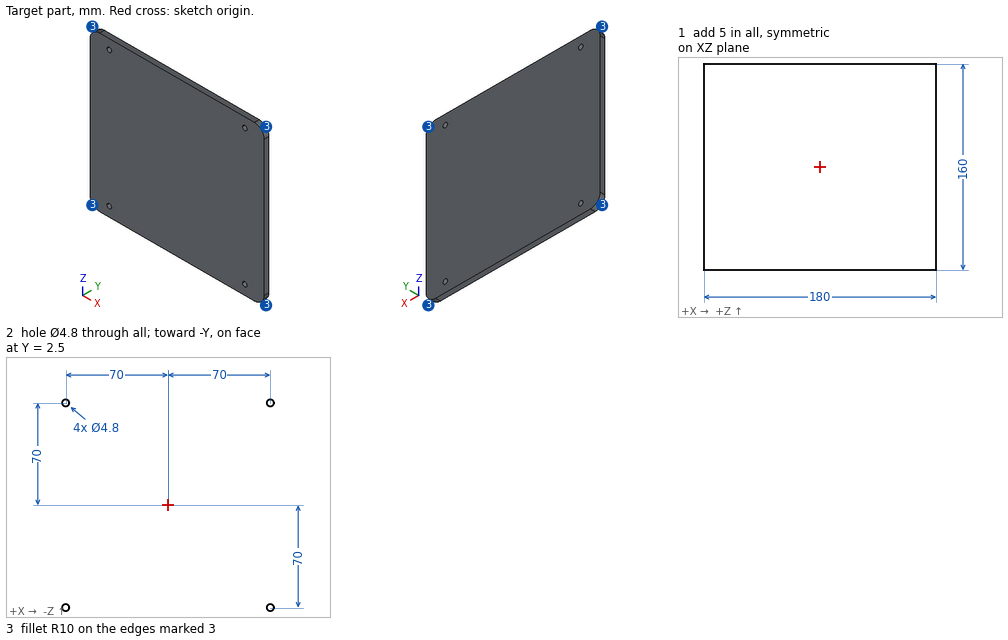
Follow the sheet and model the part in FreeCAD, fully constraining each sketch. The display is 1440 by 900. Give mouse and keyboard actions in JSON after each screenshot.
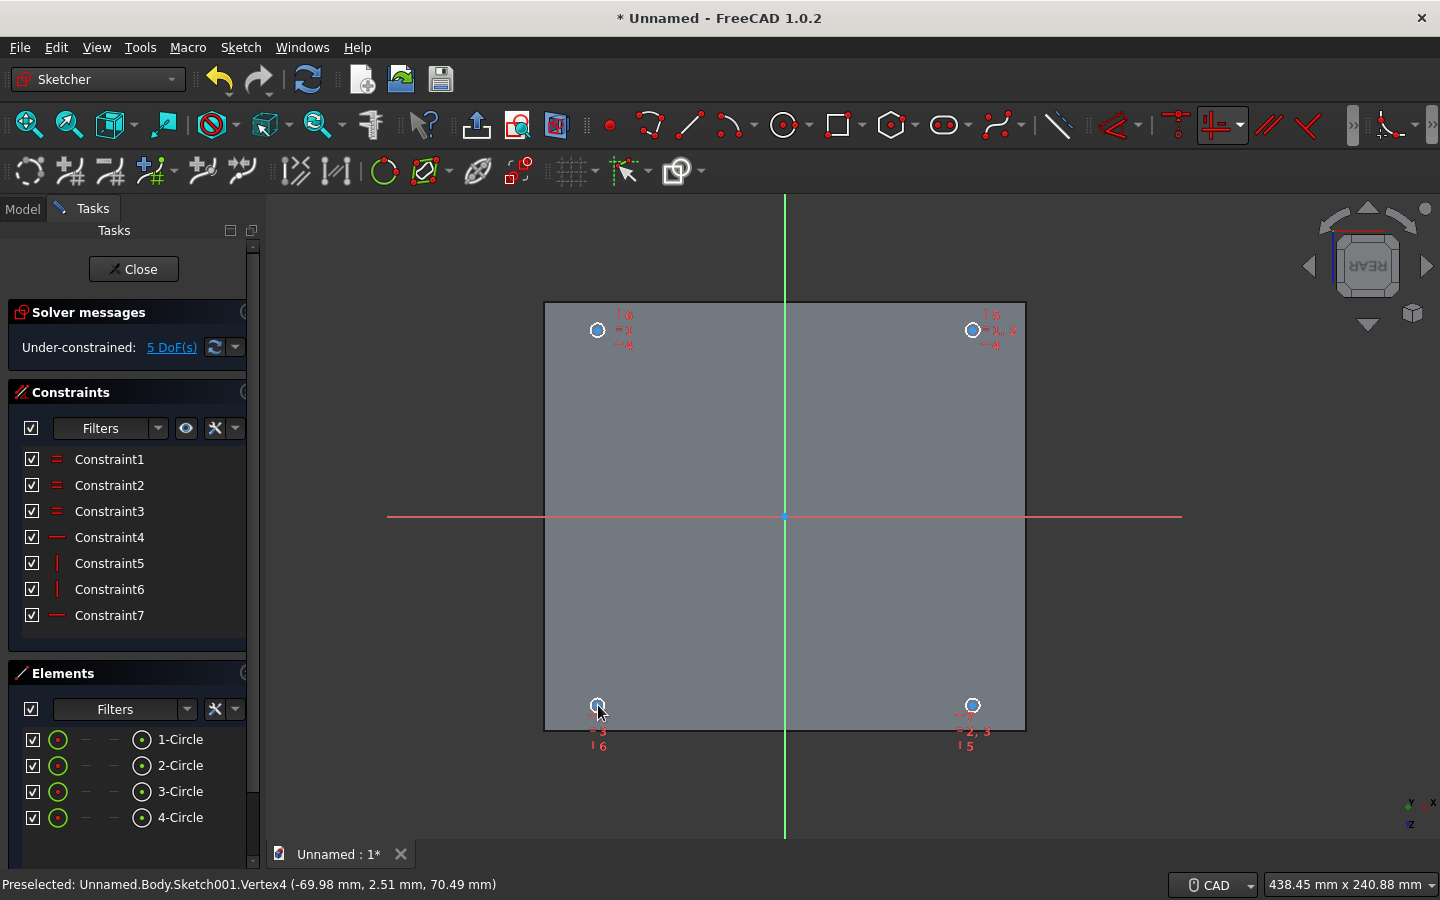
{"action": "left_click", "coordinate": [1114, 126]}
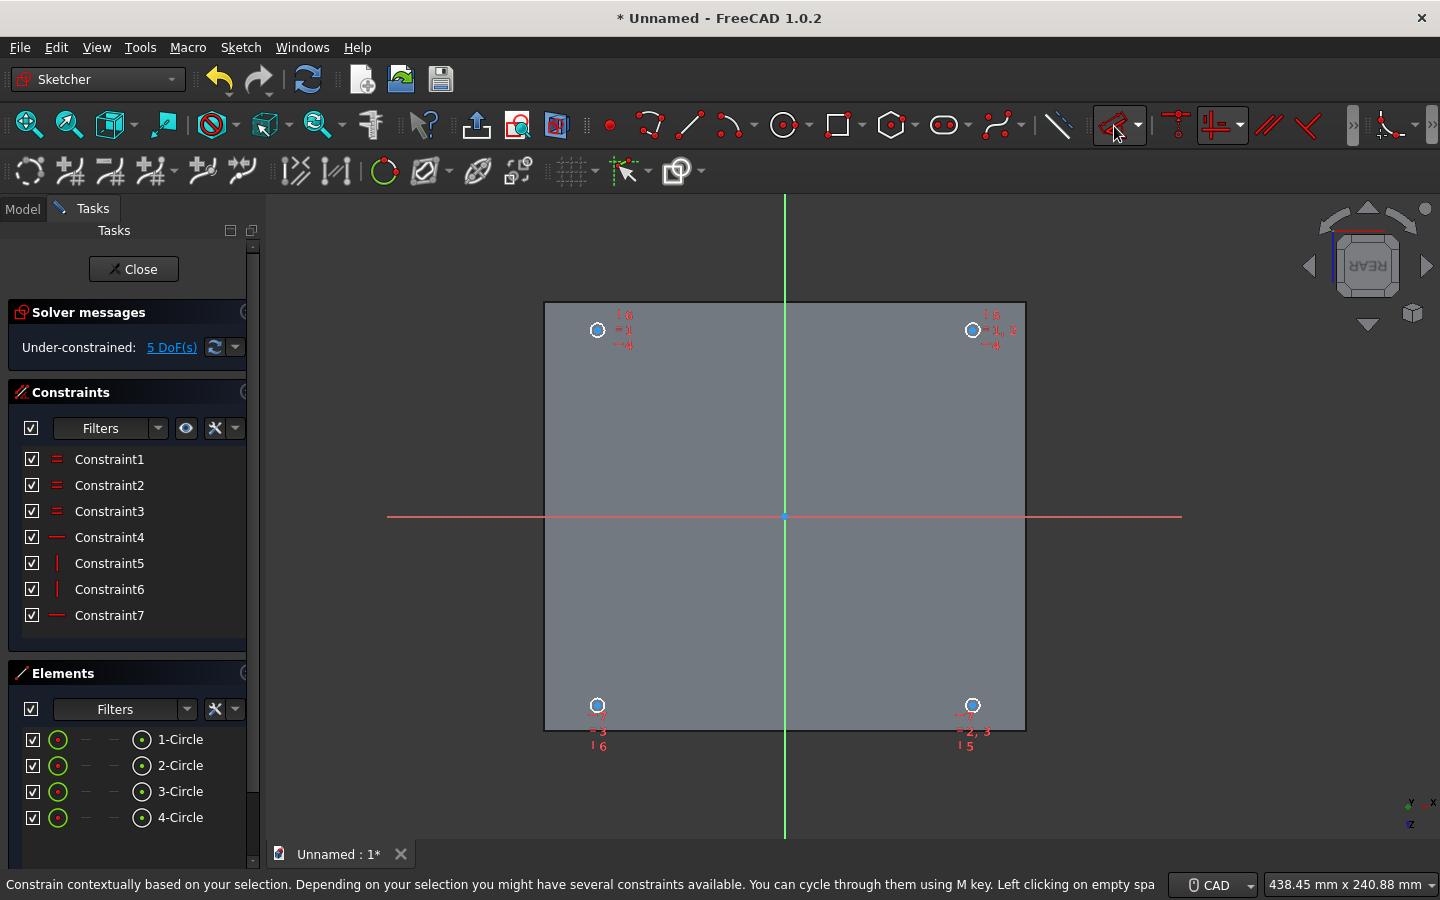
{"action": "scroll", "coordinate": [602, 325], "scroll_direction": "up", "scroll_amount": 6}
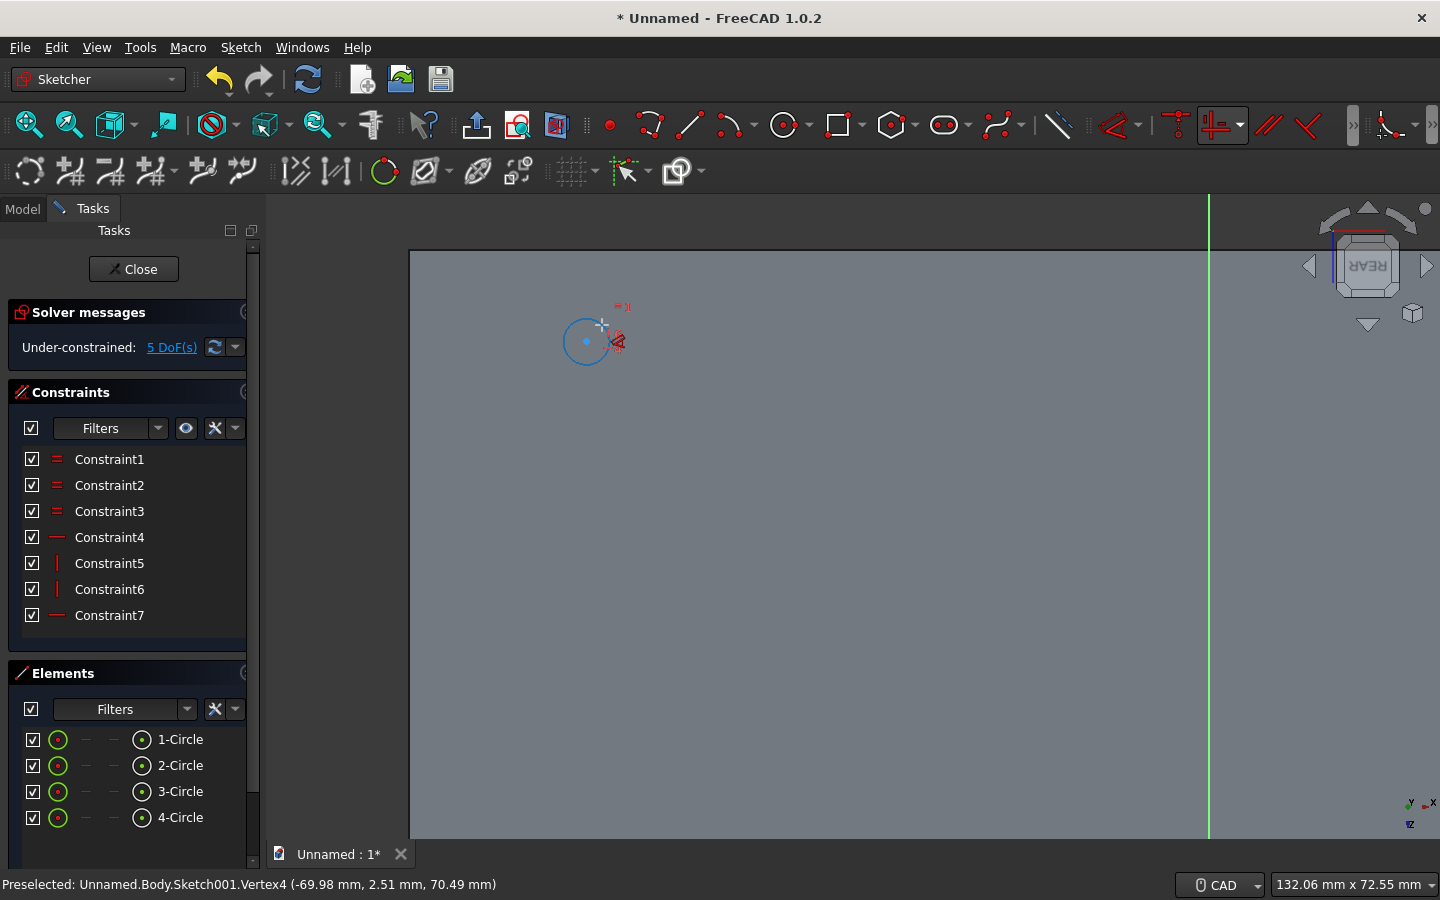
{"action": "left_click", "coordinate": [603, 325]}
{"action": "left_click", "coordinate": [625, 302]}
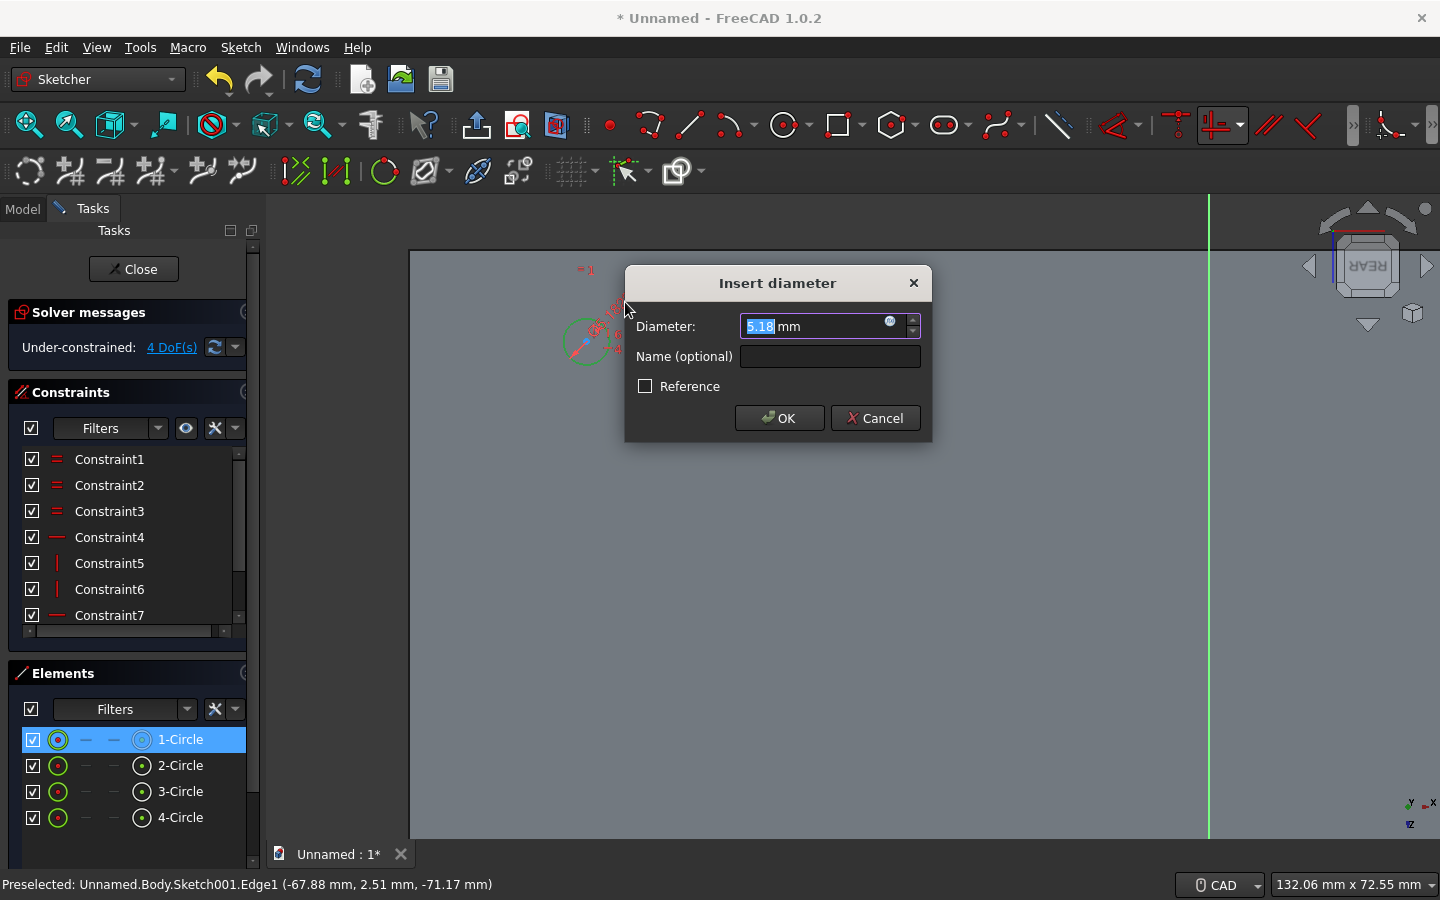
{"action": "type", "text": "4.8"}
{"action": "key", "text": "Return"}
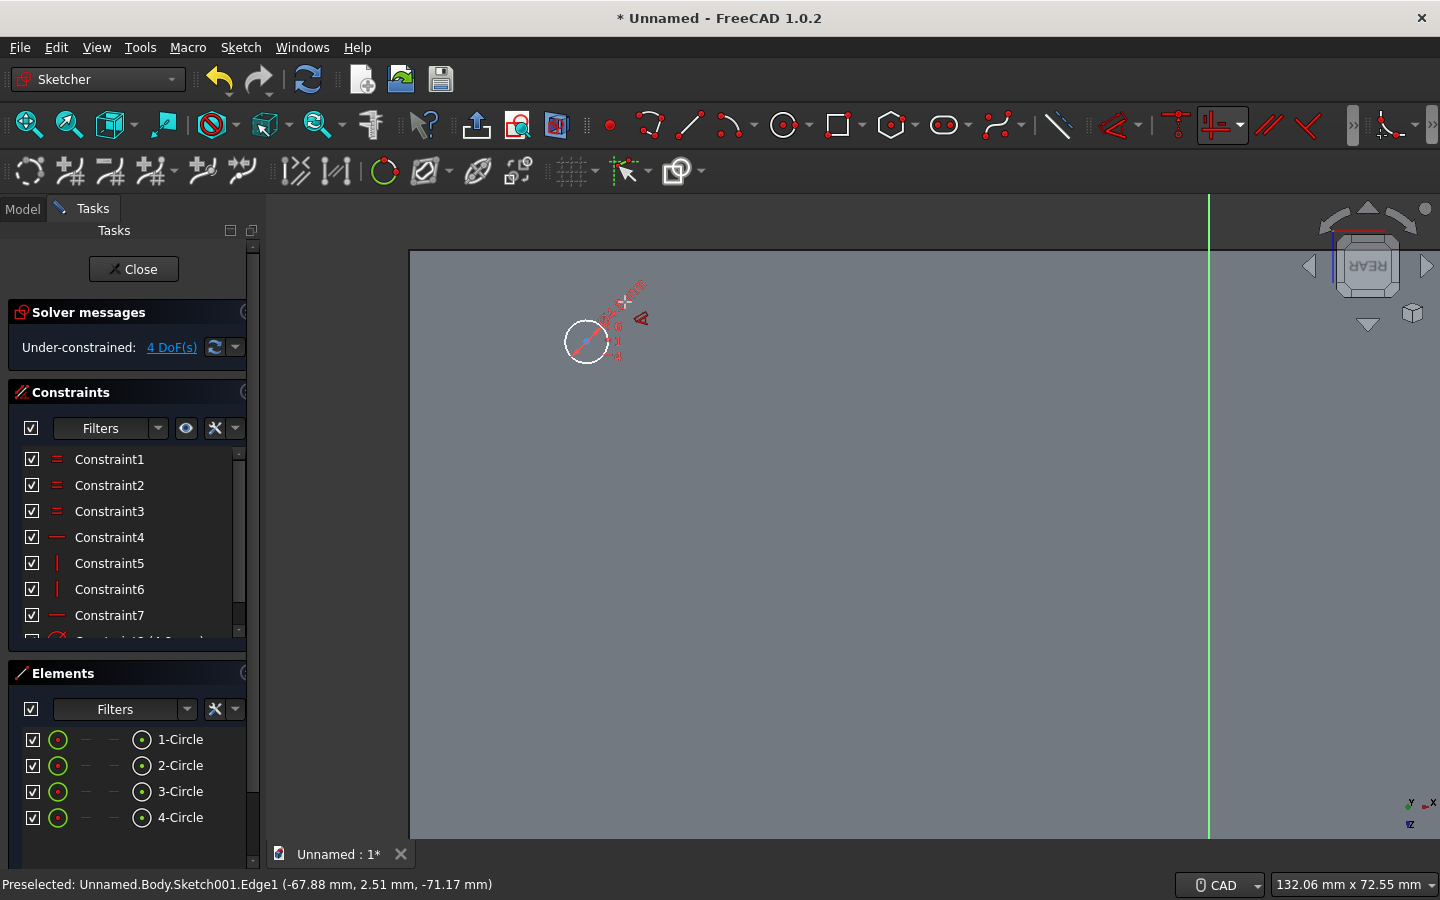
{"action": "left_click", "coordinate": [587, 342]}
{"action": "left_click", "coordinate": [898, 308]}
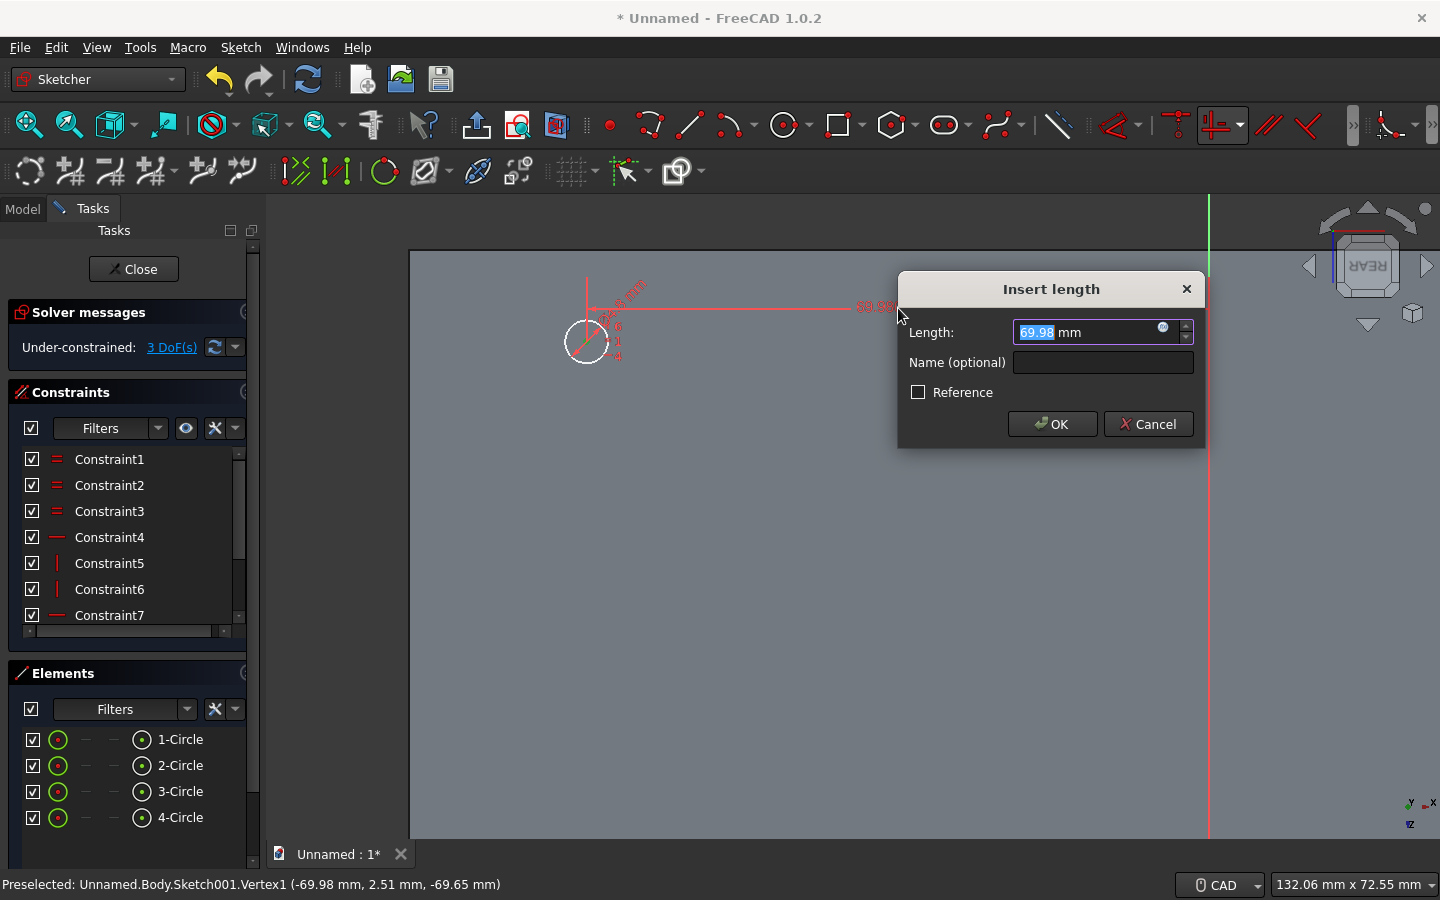
{"action": "type", "text": "70"}
{"action": "key", "text": "Return"}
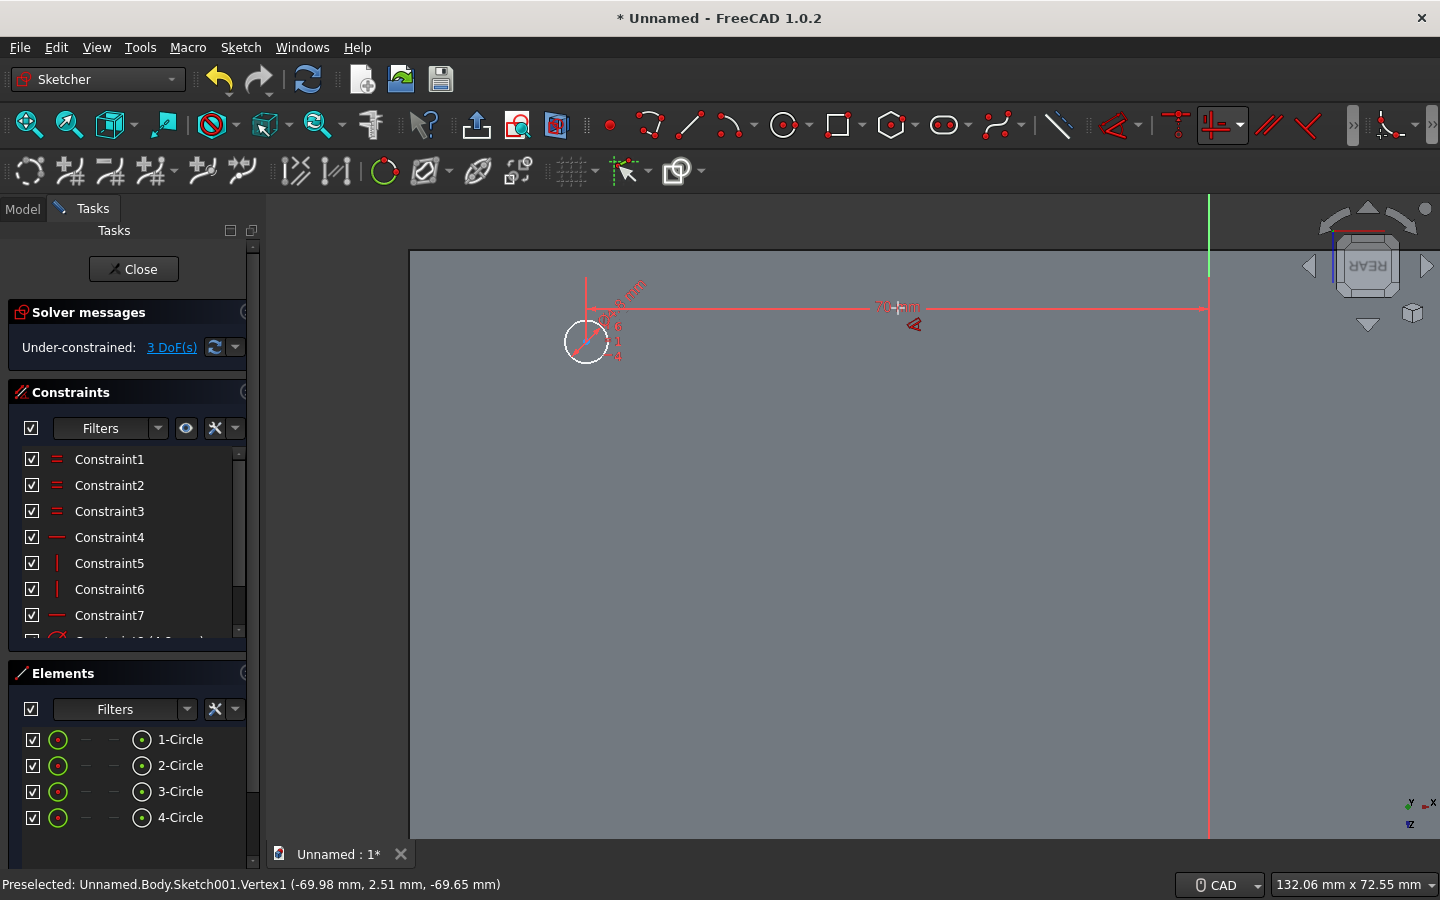
{"action": "left_click", "coordinate": [586, 342]}
{"action": "left_click", "coordinate": [552, 576]}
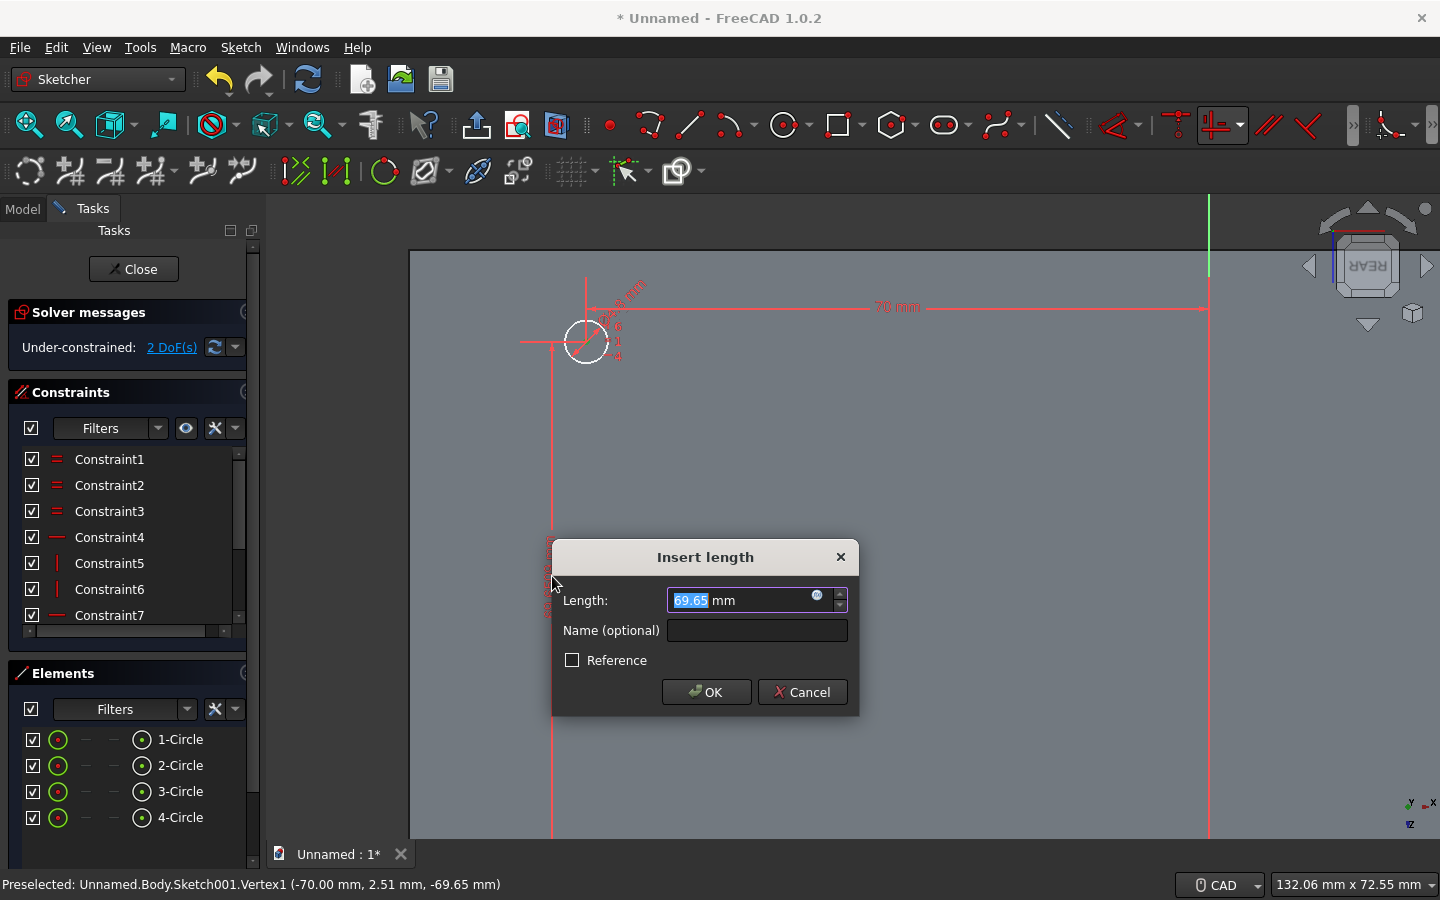
{"action": "type", "text": "70"}
{"action": "key", "text": "Return"}